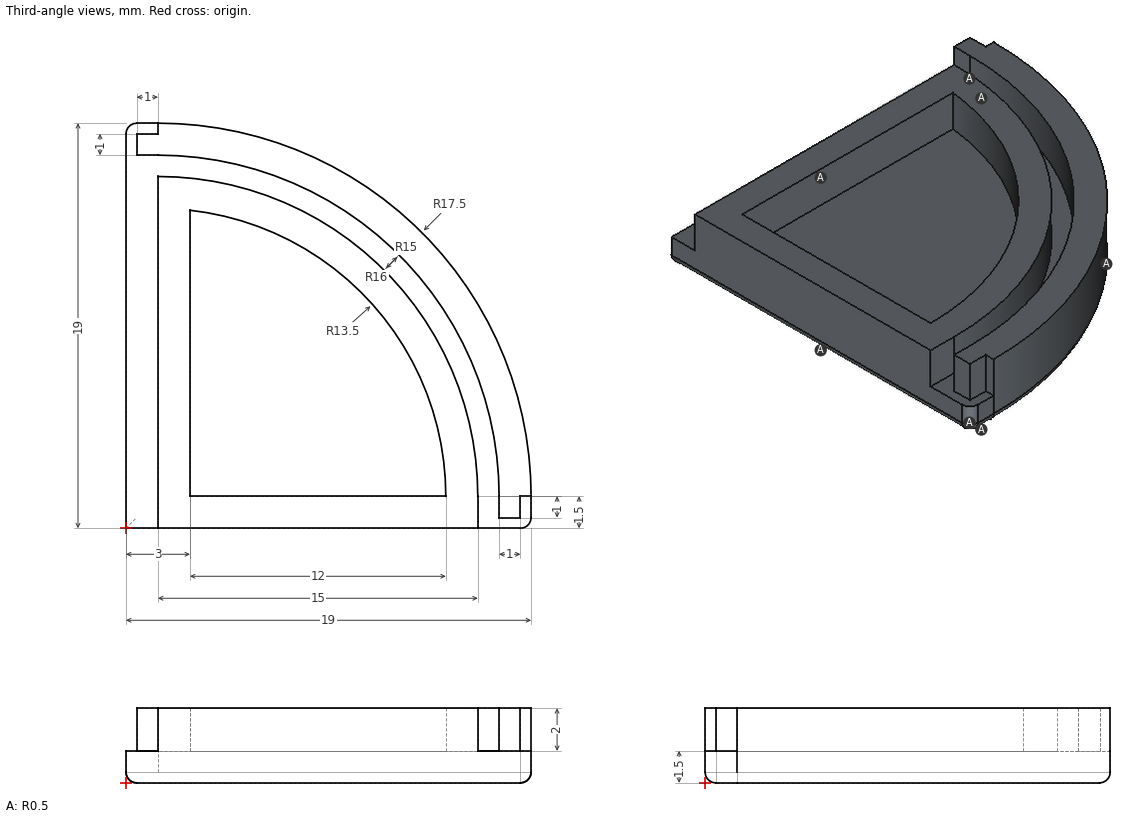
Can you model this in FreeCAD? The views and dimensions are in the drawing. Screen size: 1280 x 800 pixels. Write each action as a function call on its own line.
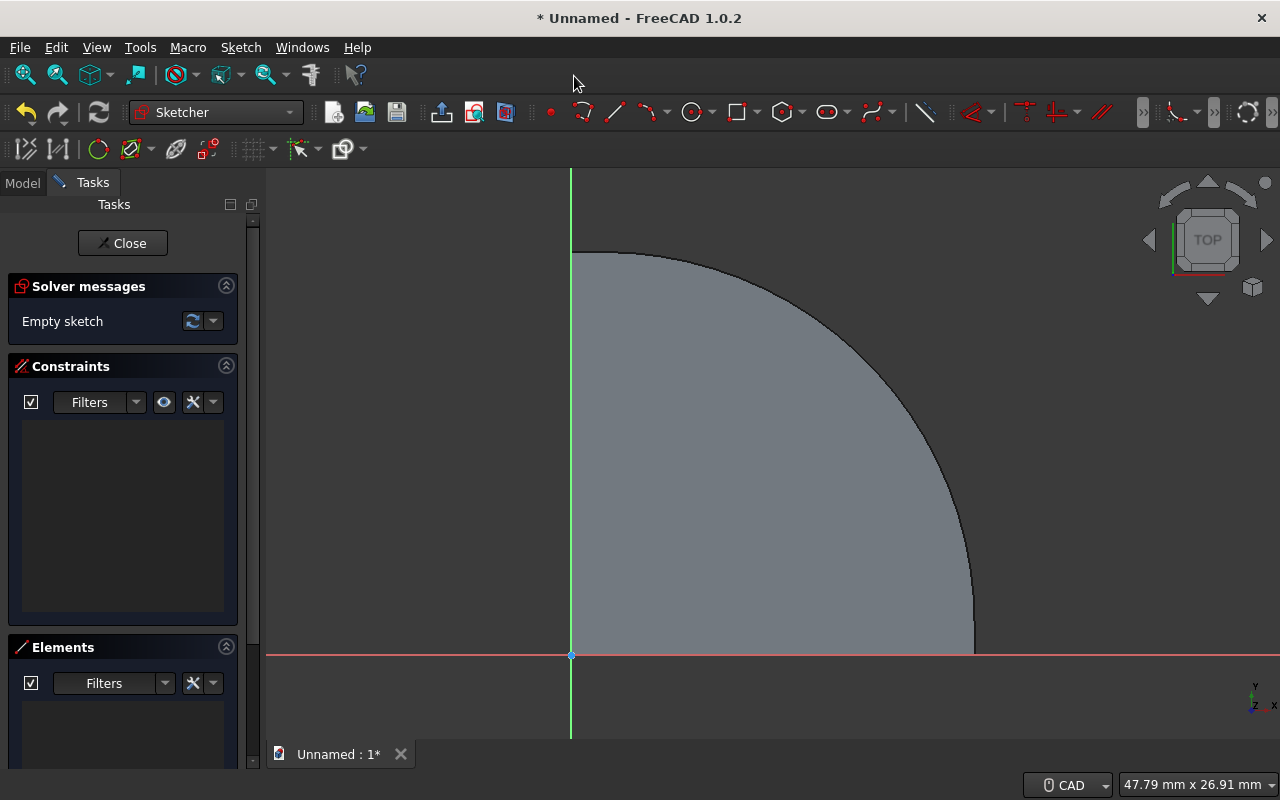
key(g)
key(m)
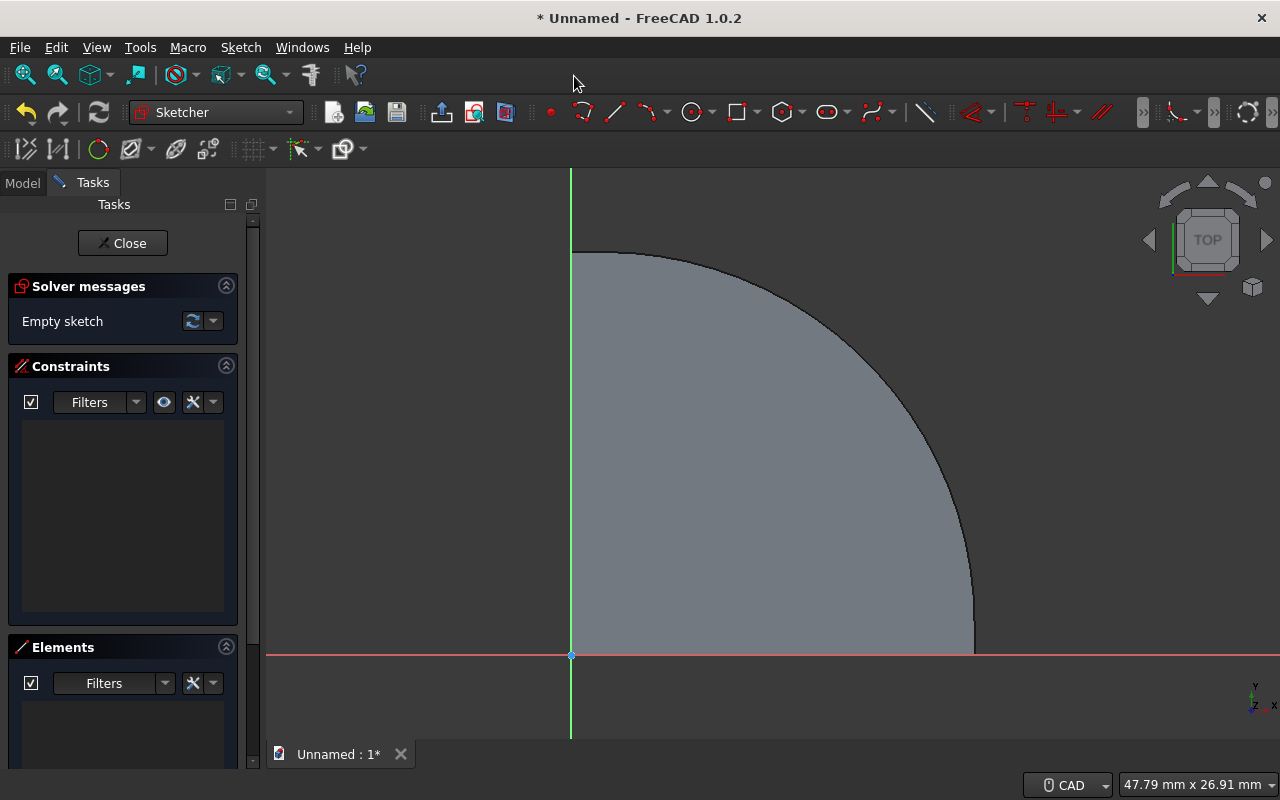
click(603, 252)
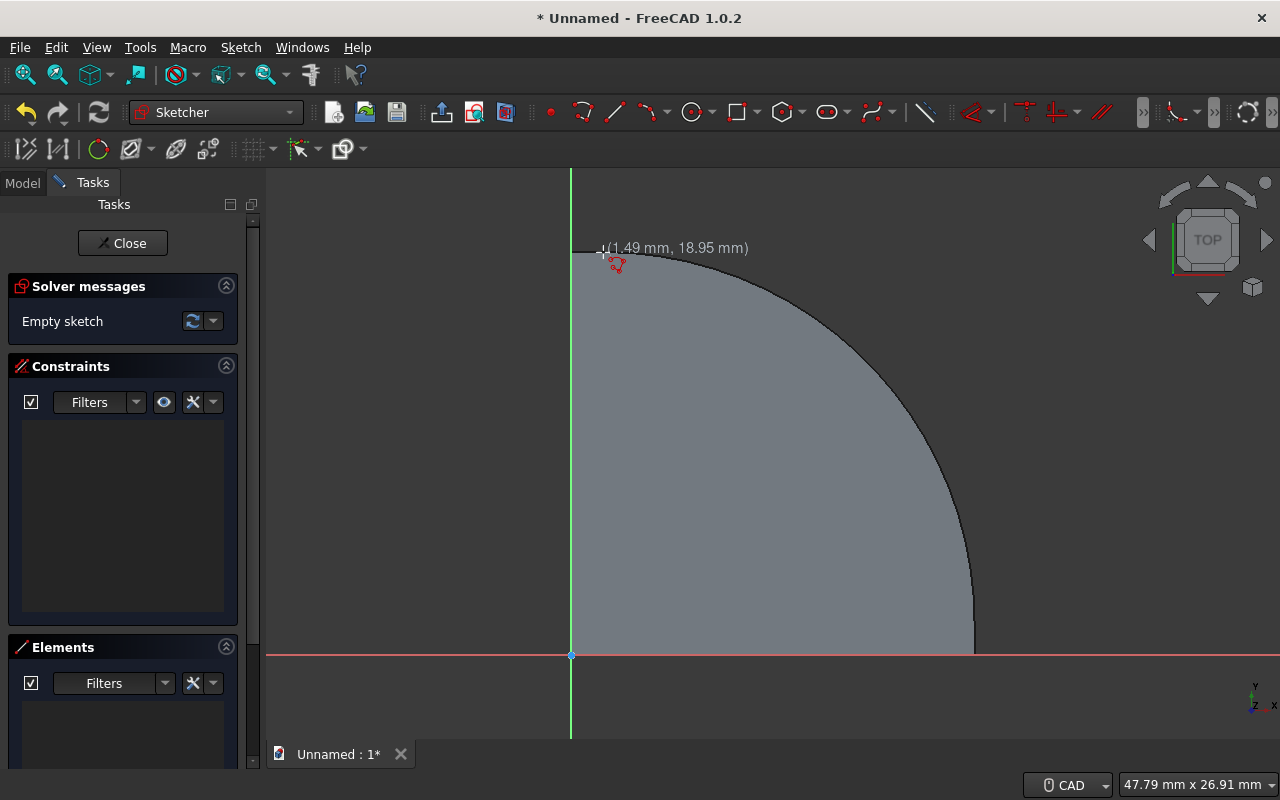
scroll(603, 263, up, 3)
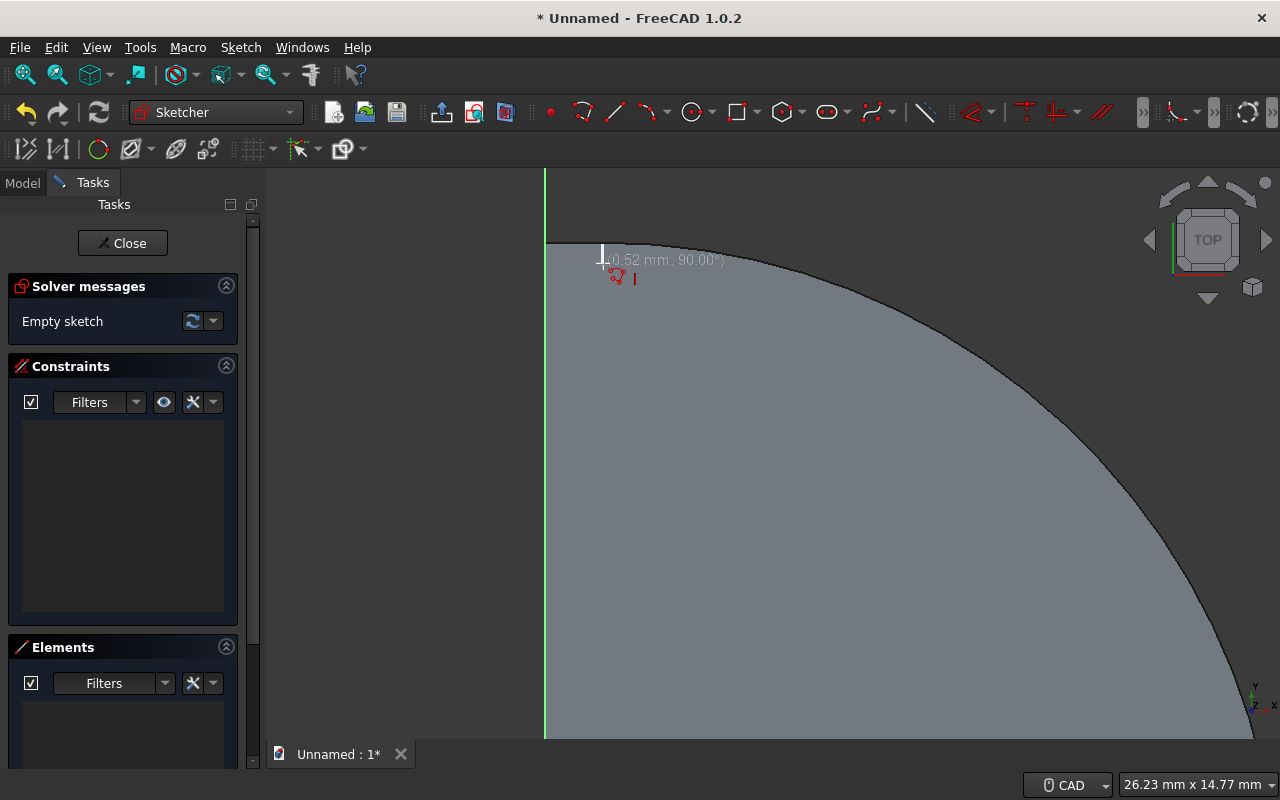
click(603, 262)
click(565, 262)
click(565, 301)
click(603, 301)
right_click(603, 301)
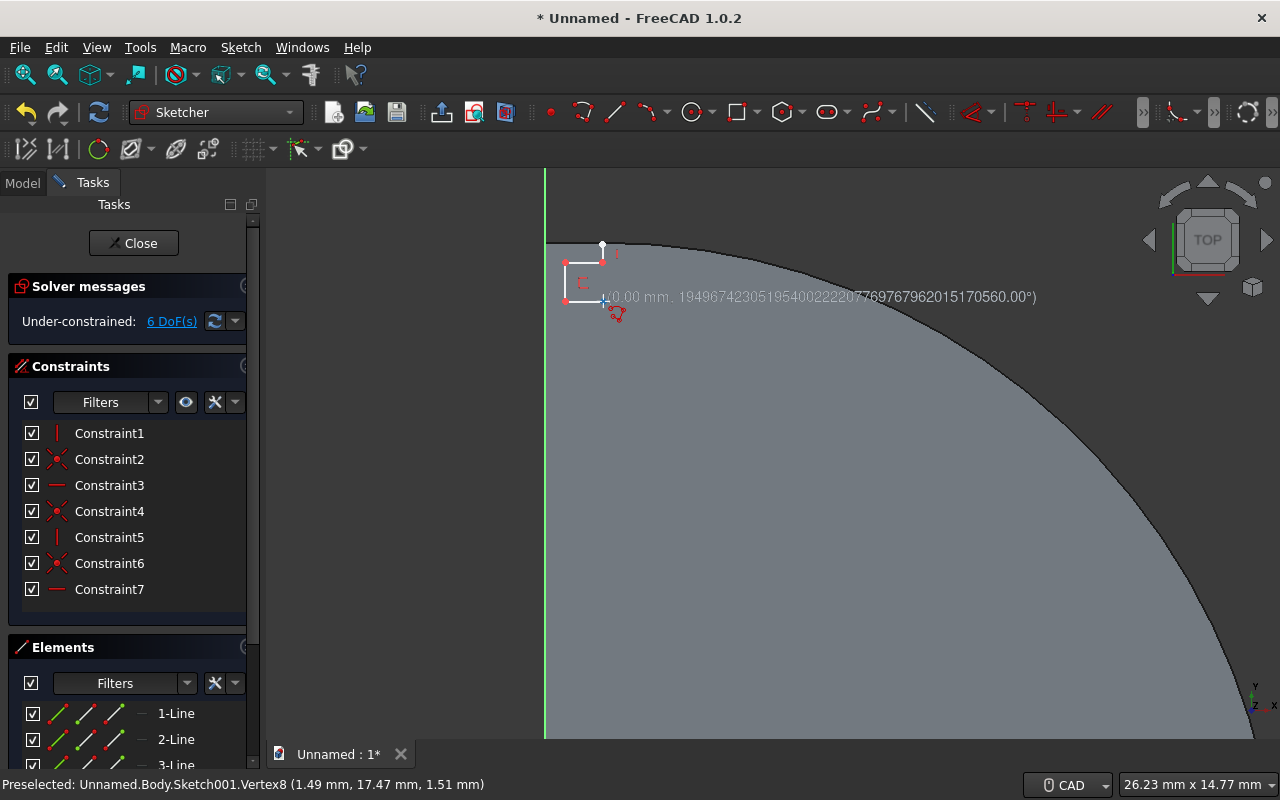
scroll(535, 326, down, 4)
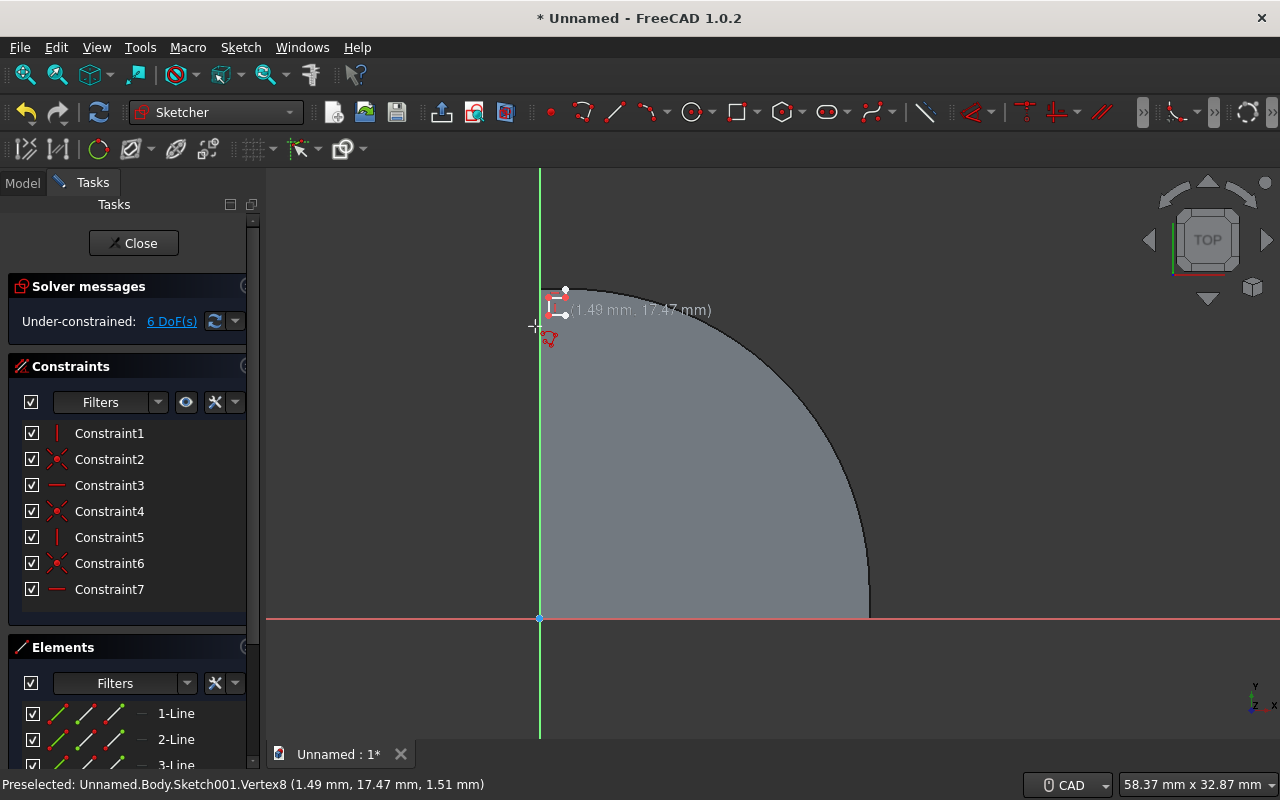
click(844, 593)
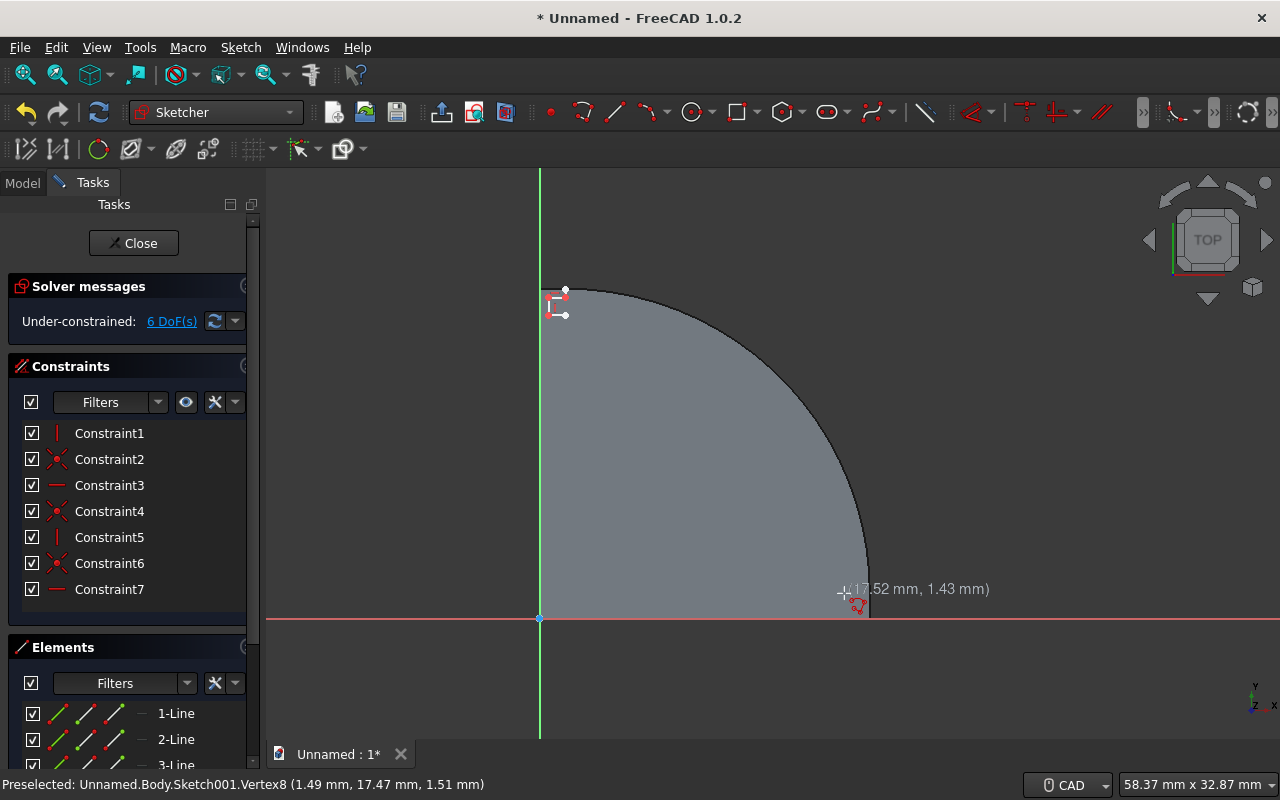
scroll(844, 610, up, 4)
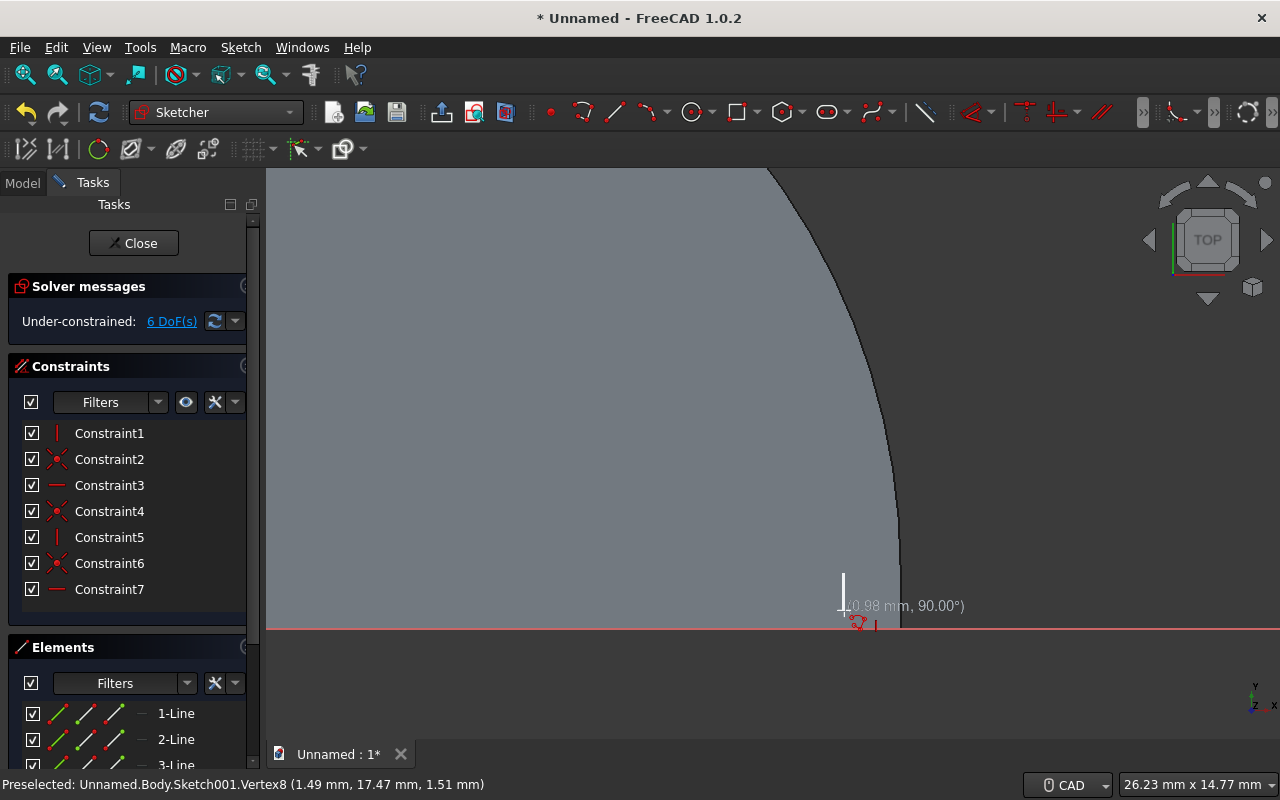
click(843, 609)
click(881, 609)
click(881, 571)
click(901, 571)
right_click(901, 571)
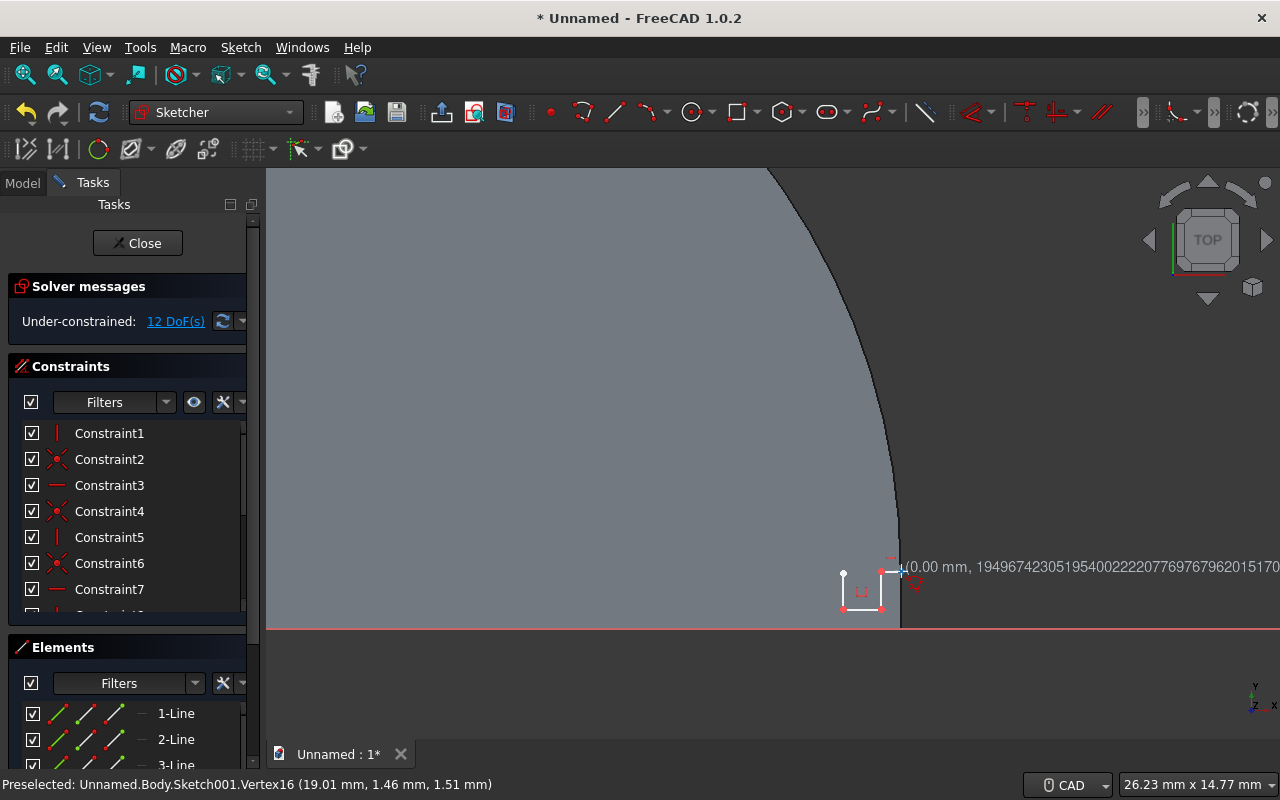
click(648, 112)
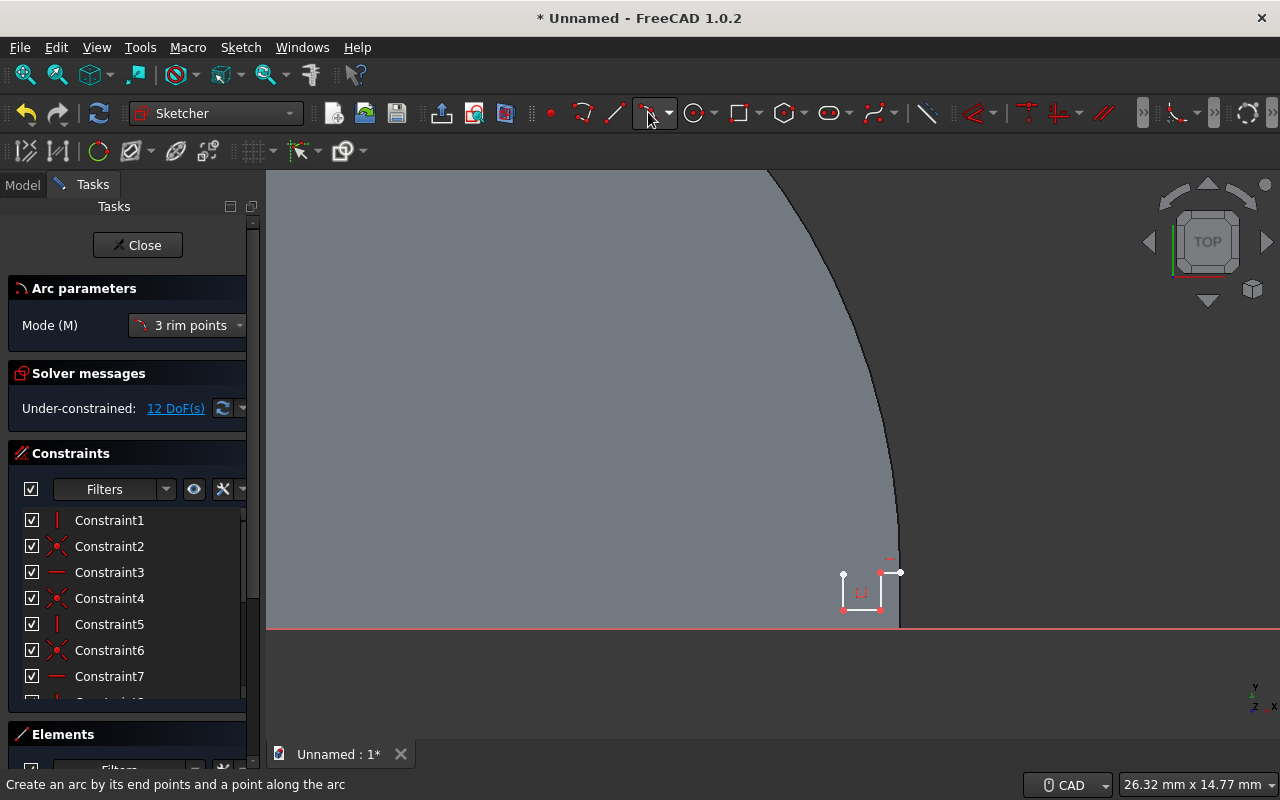
scroll(843, 611, down, 4)